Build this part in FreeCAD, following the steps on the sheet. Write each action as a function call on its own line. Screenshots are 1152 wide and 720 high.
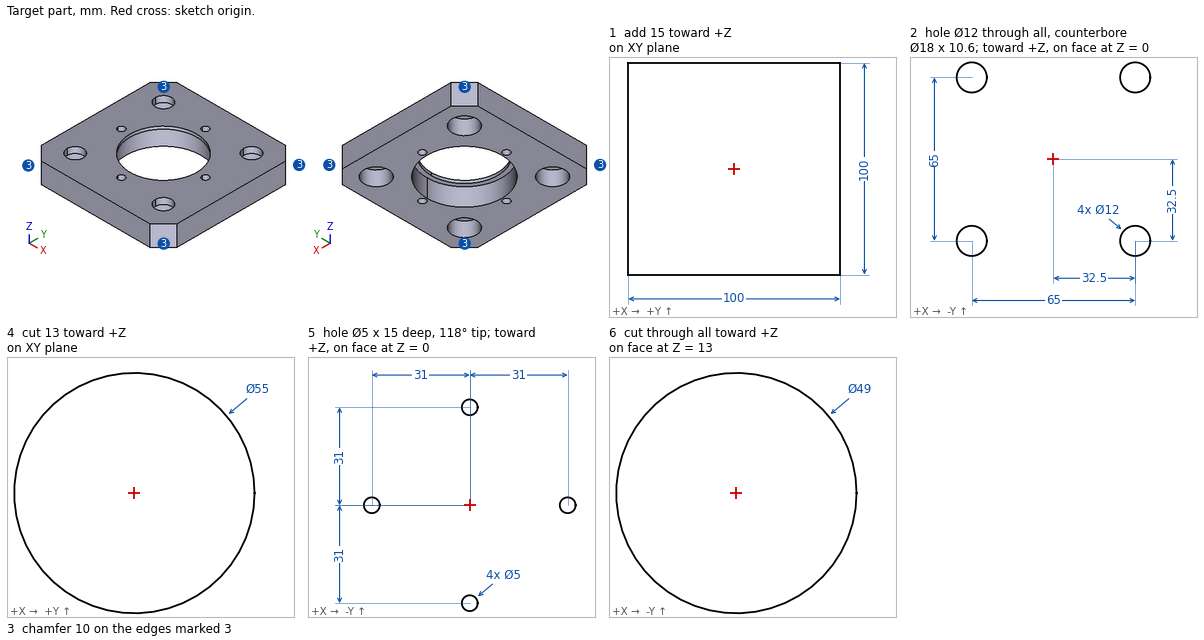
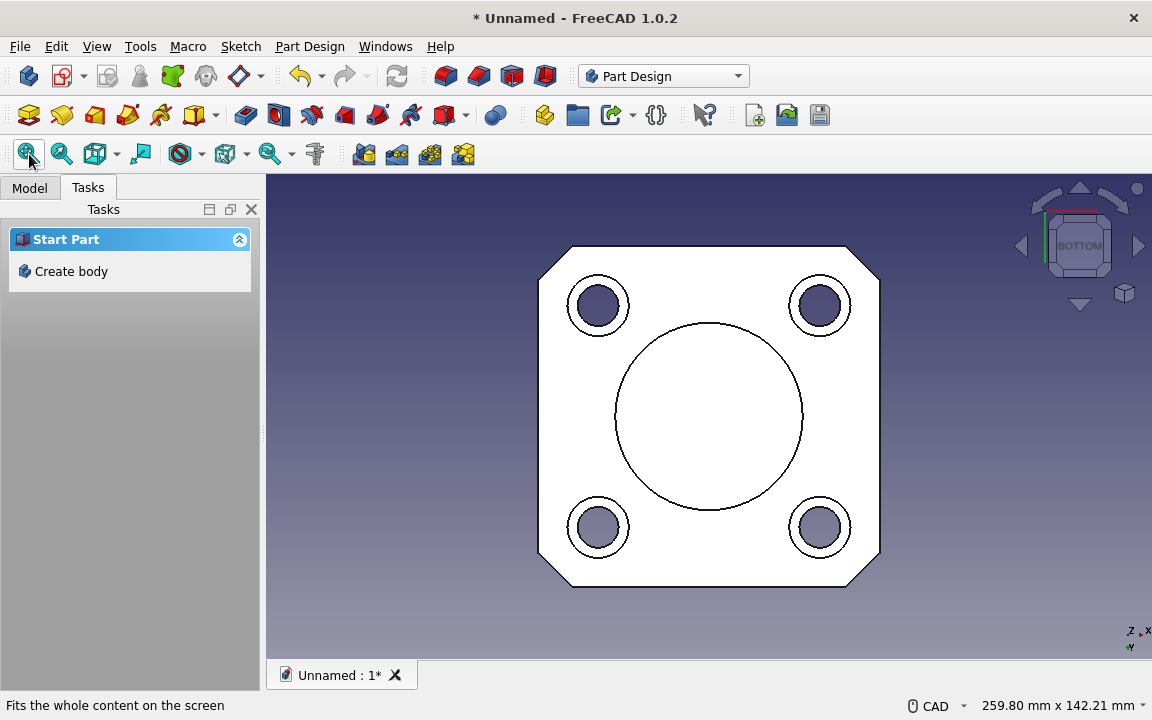
click(758, 269)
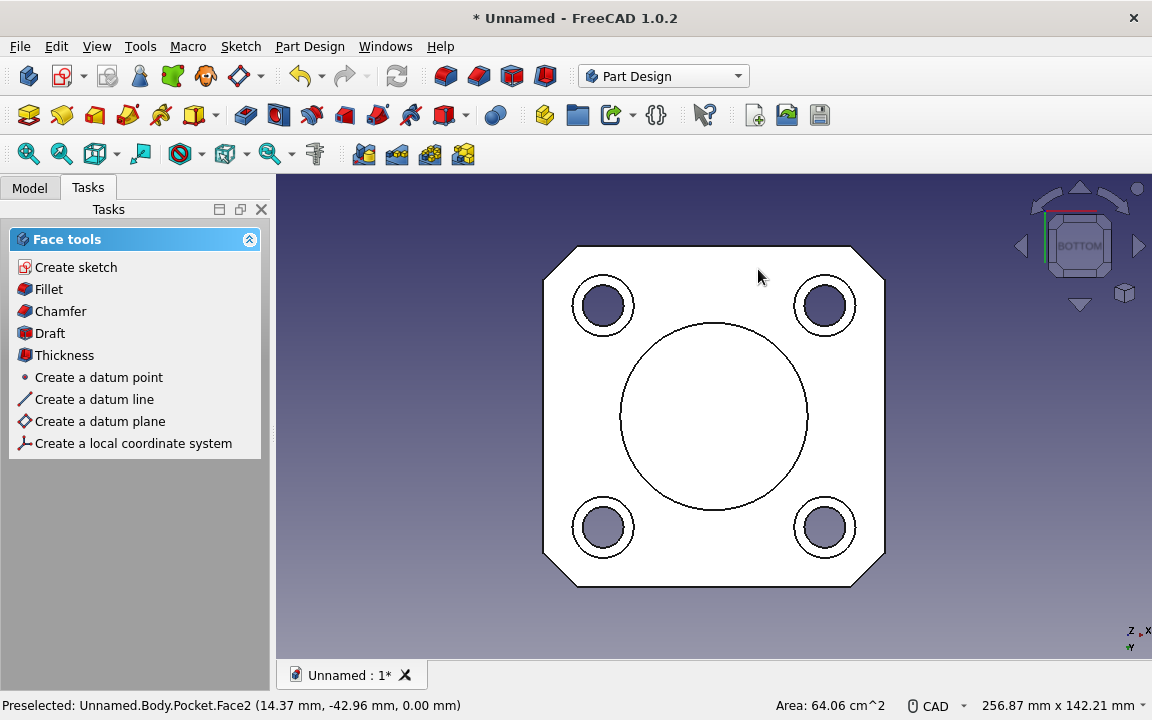
click(62, 76)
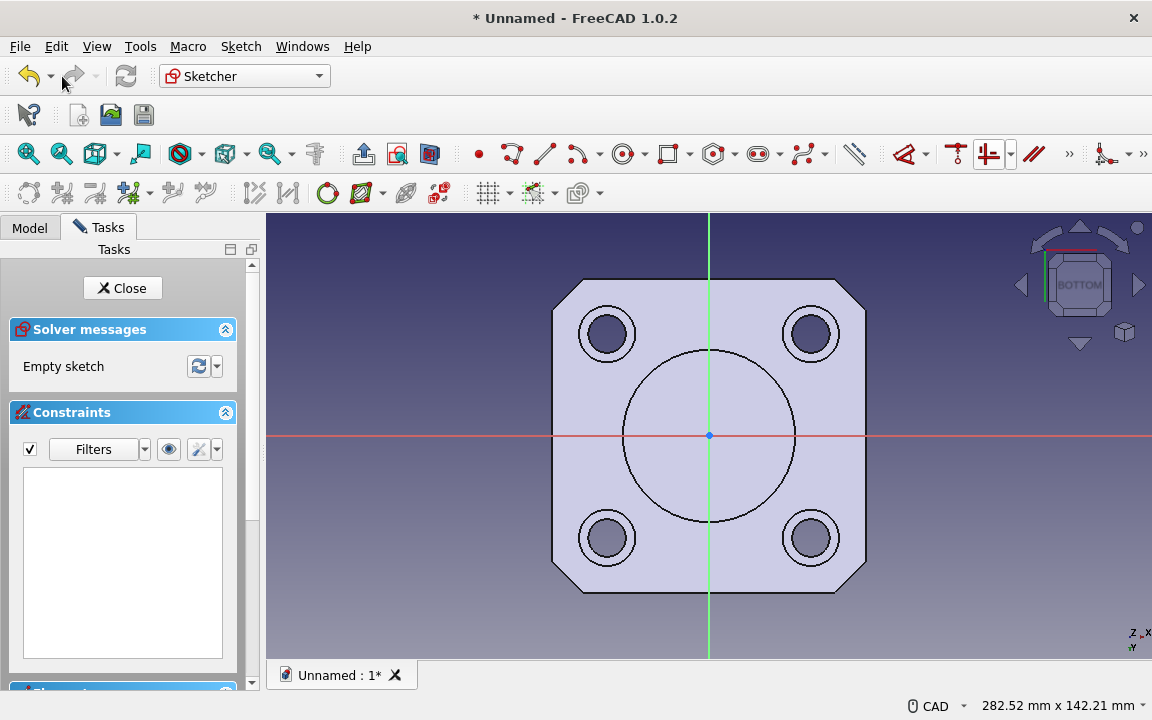
click(622, 154)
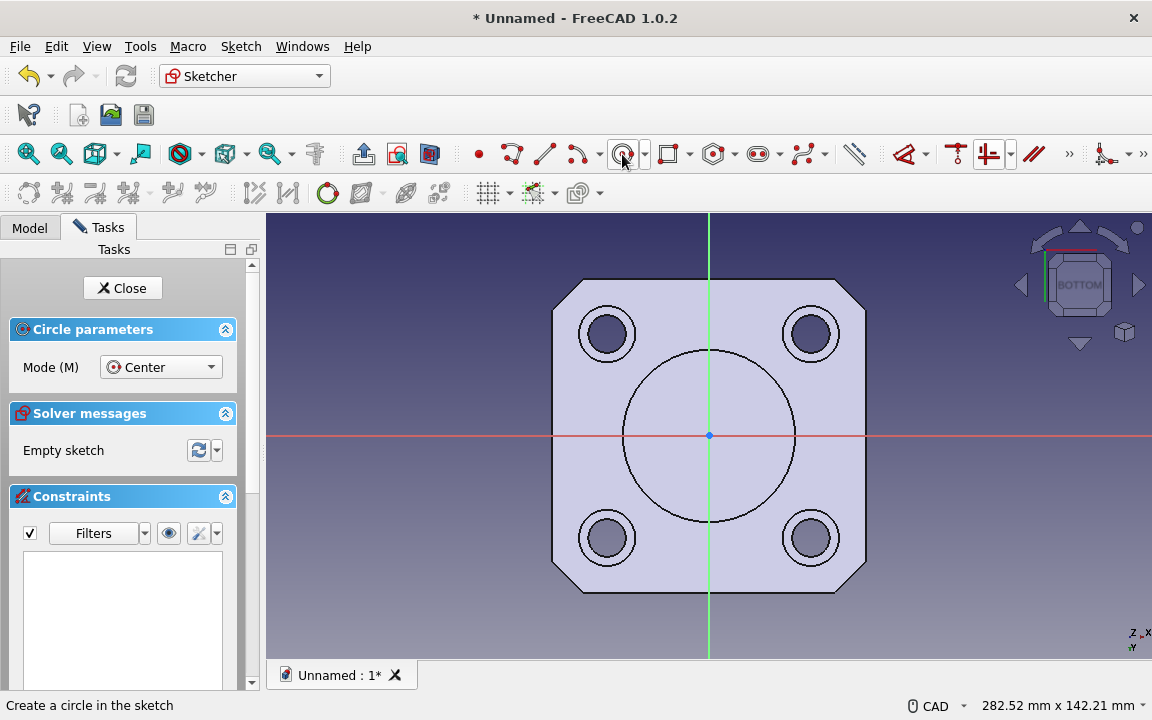
scroll(709, 533, up, 6)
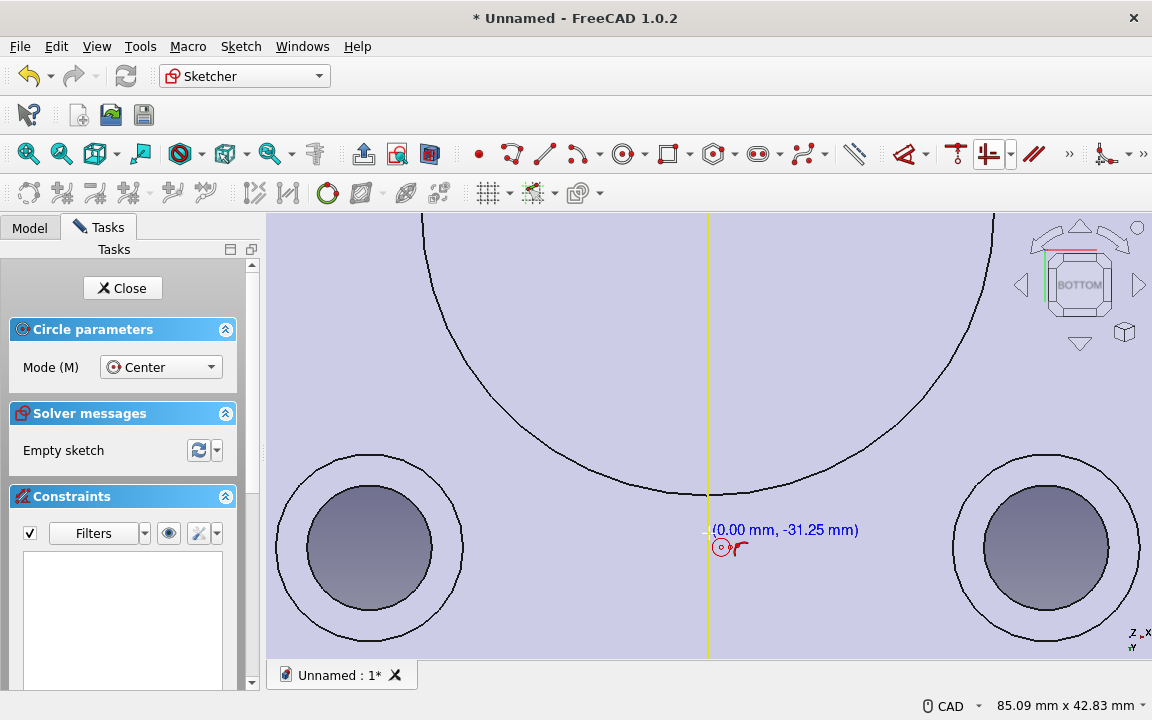
click(708, 532)
move(726, 514)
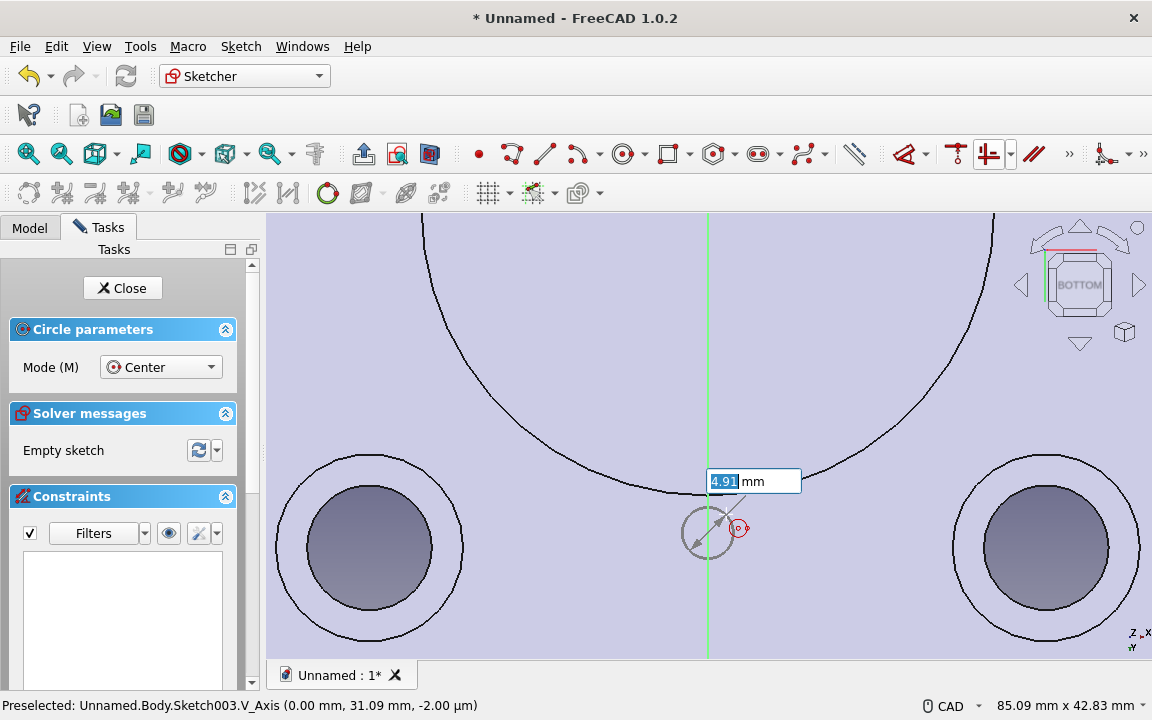
text(5)
key(Return)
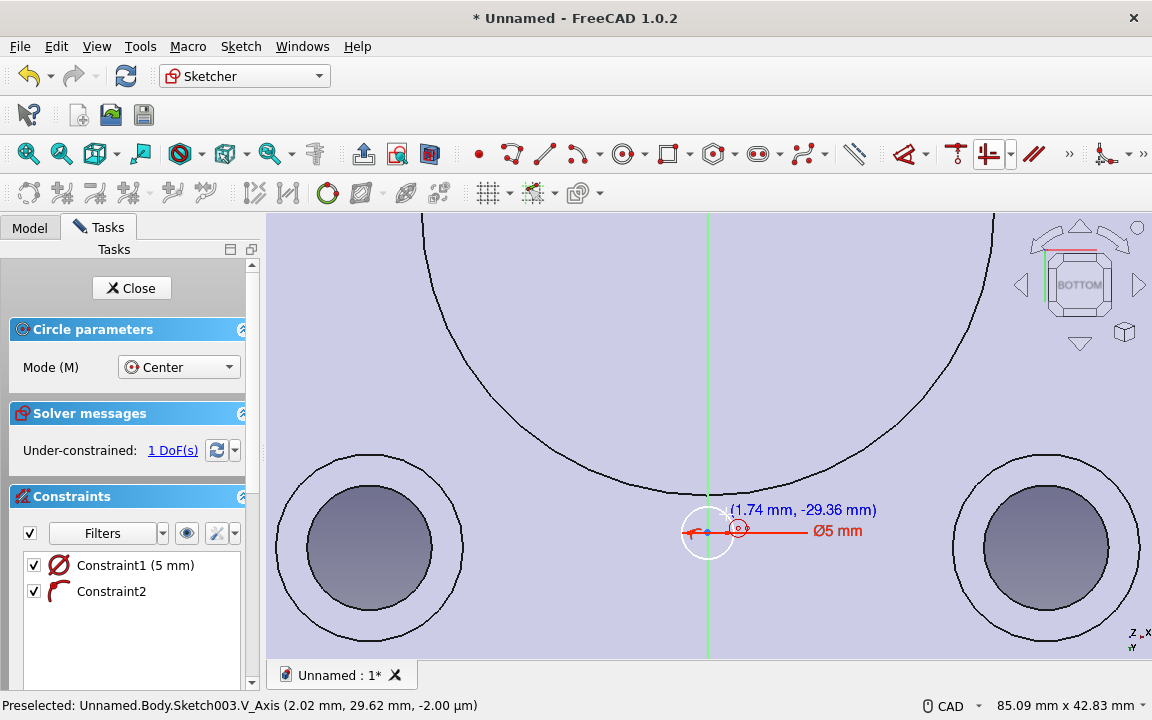
scroll(601, 568, down, 5)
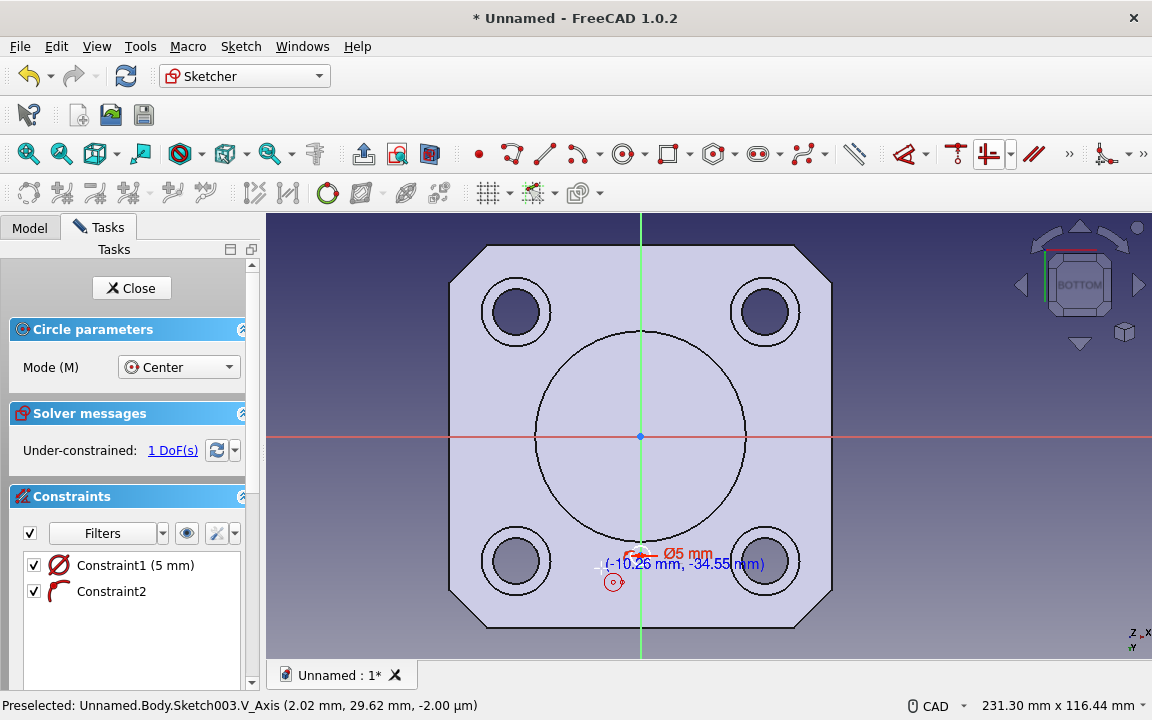
scroll(522, 437, up, 5)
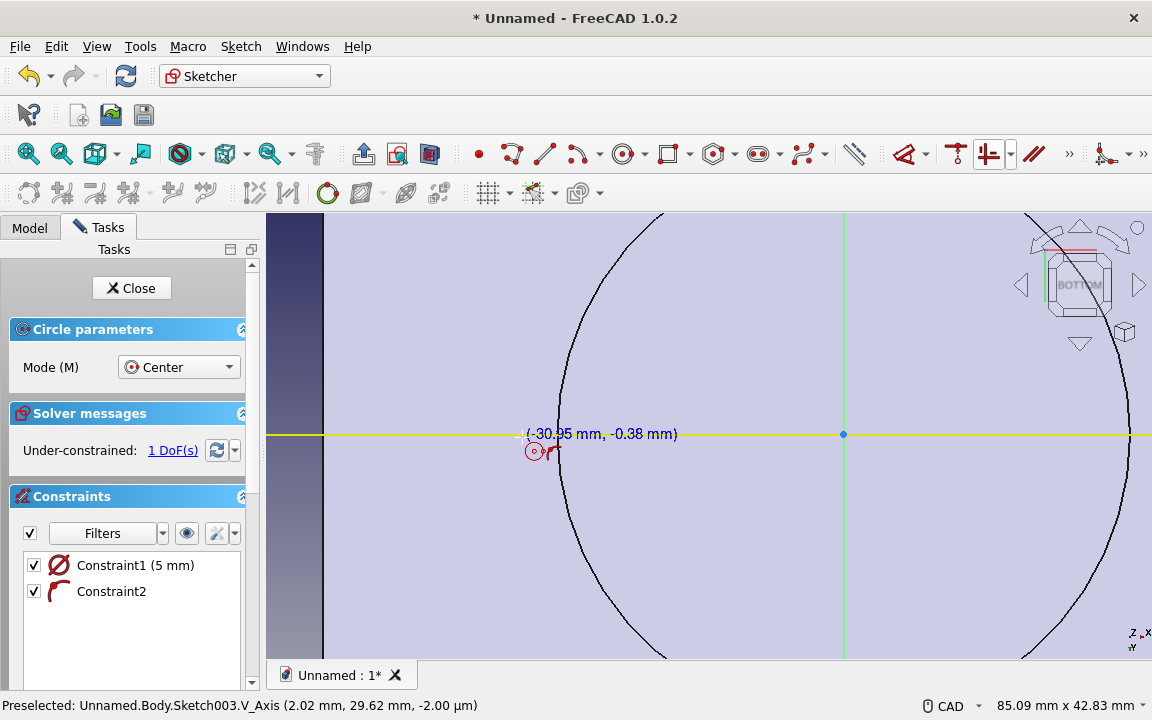
click(521, 435)
move(539, 416)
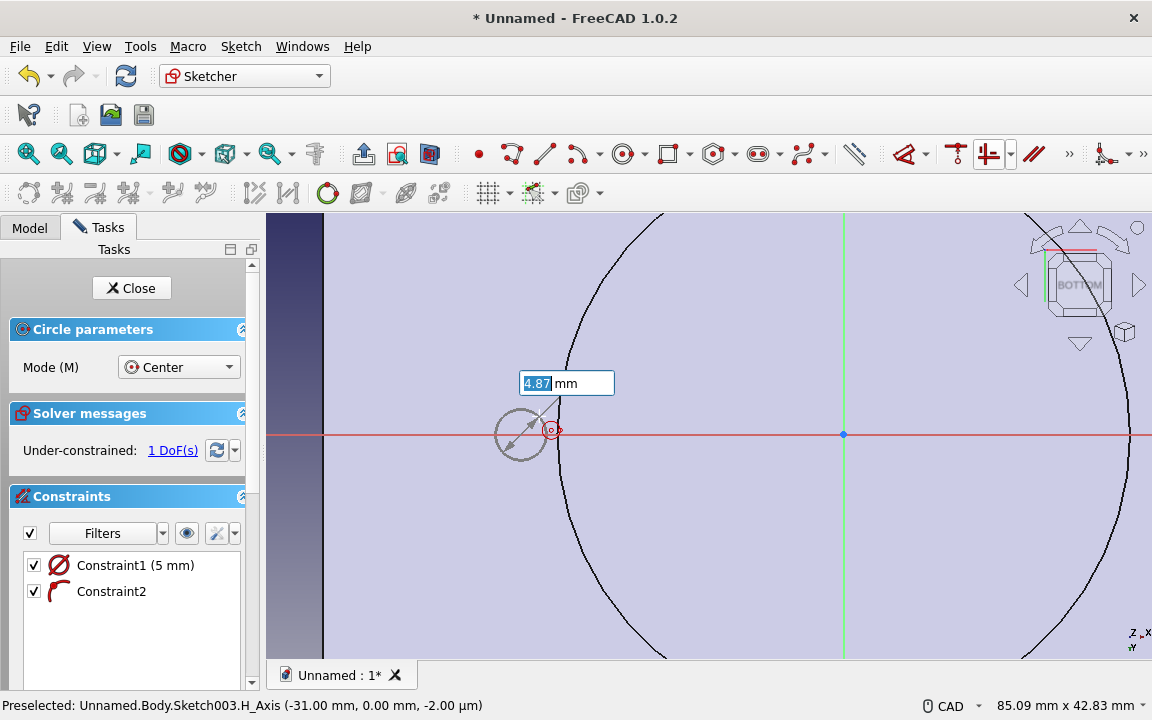
text(5)
key(Return)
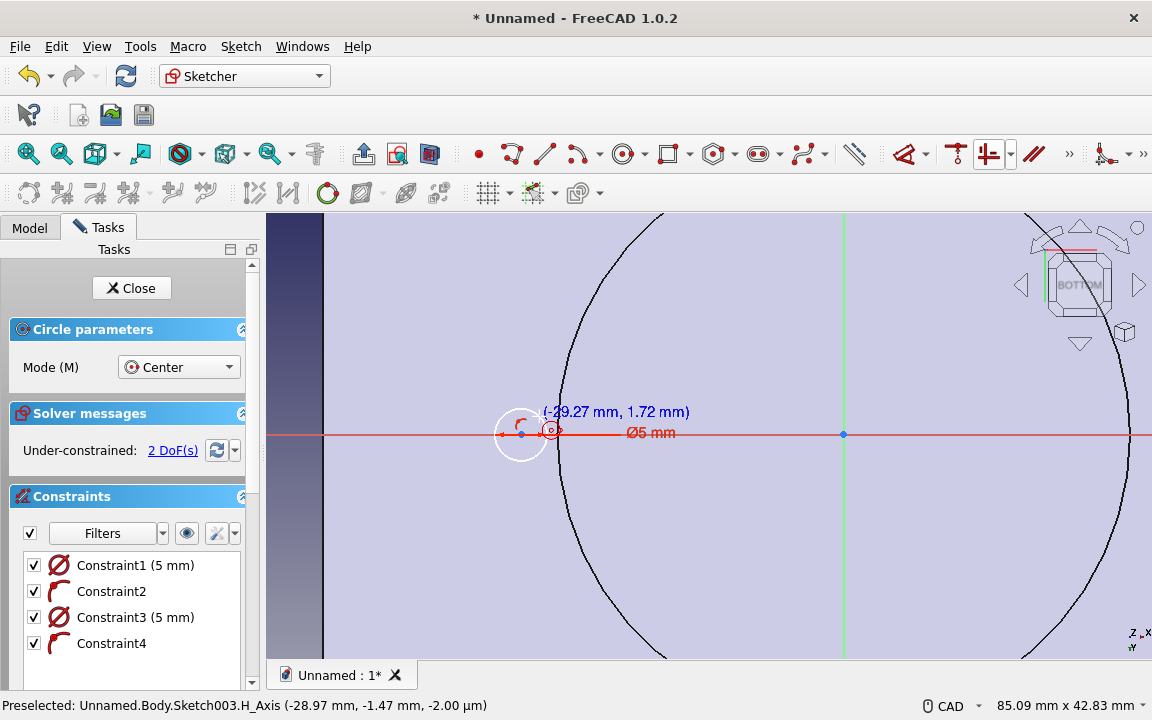
scroll(522, 437, down, 5)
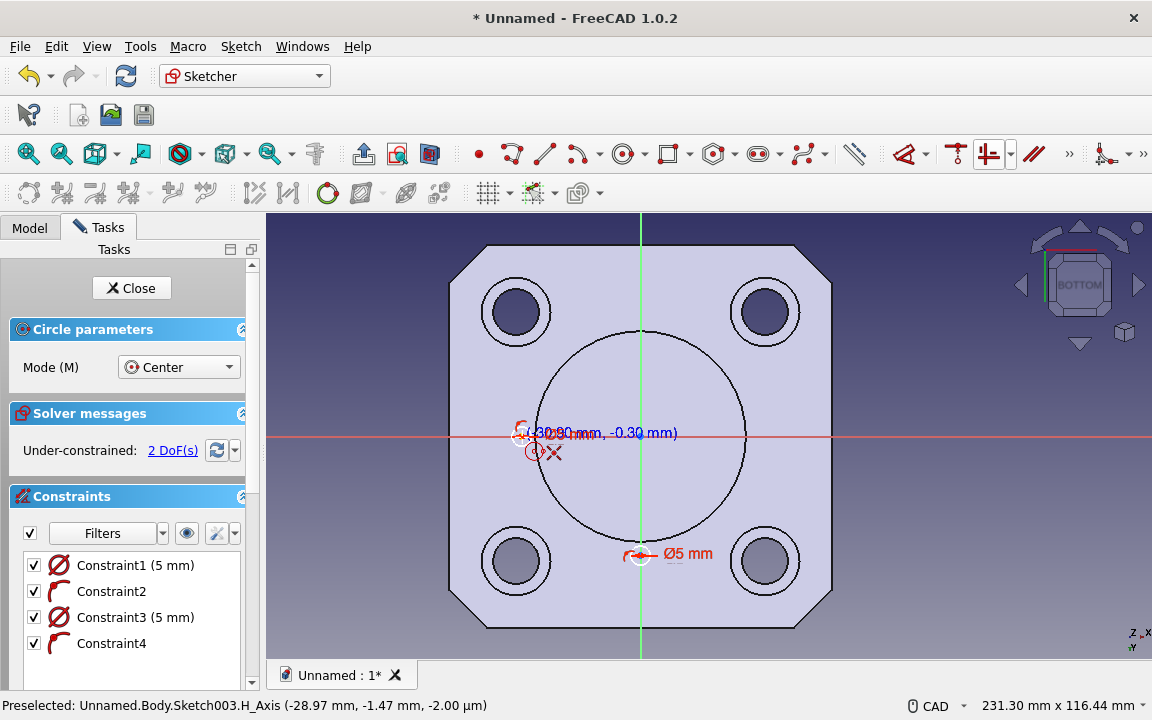
scroll(641, 318, up, 5)